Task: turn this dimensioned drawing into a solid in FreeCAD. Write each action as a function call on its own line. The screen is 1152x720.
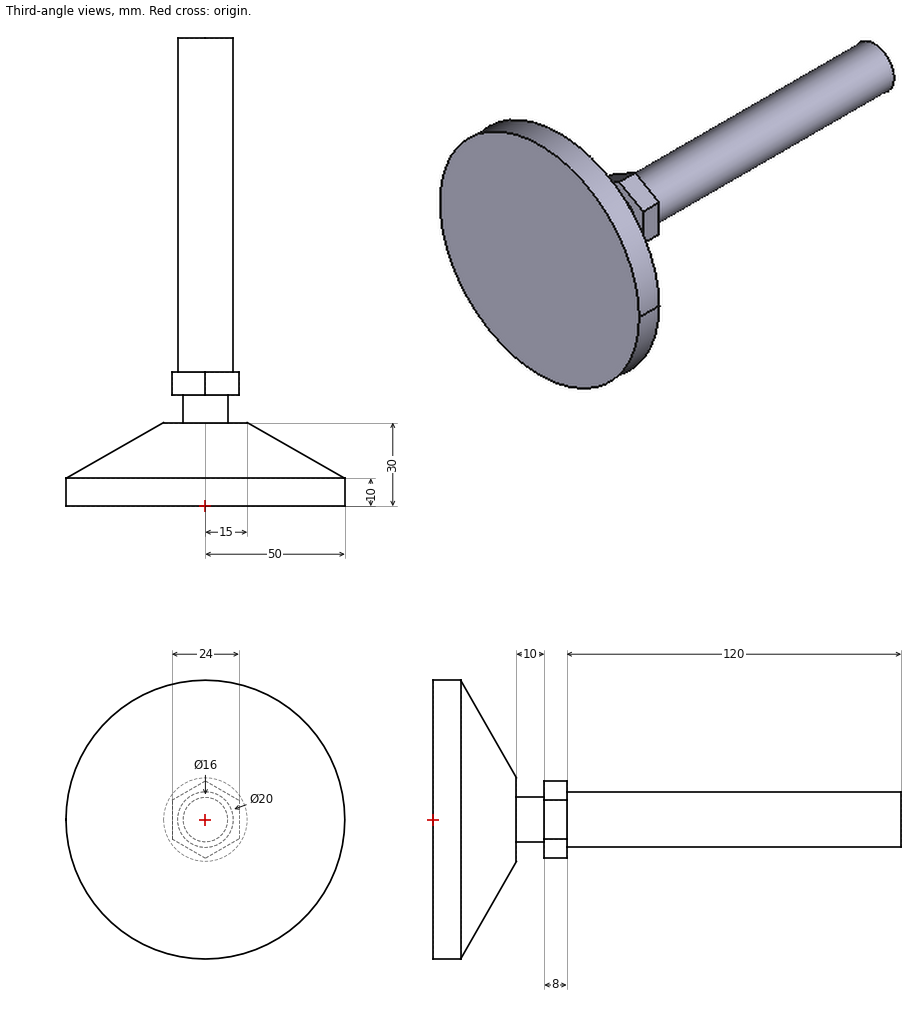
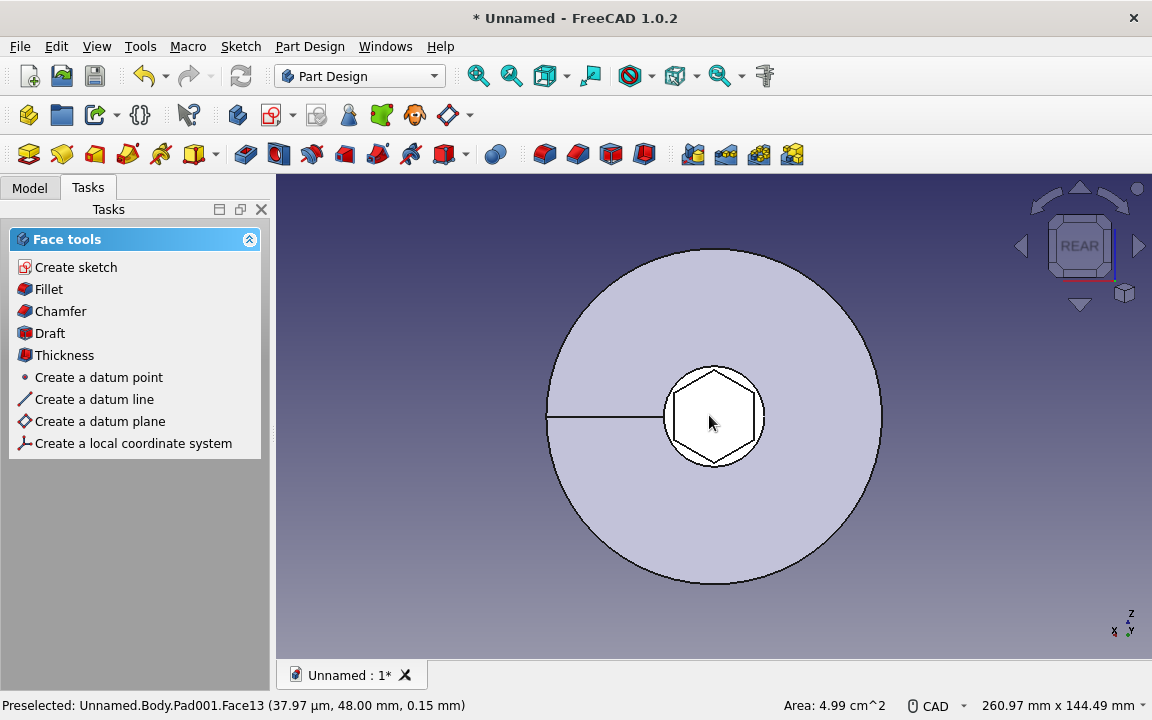
click(270, 116)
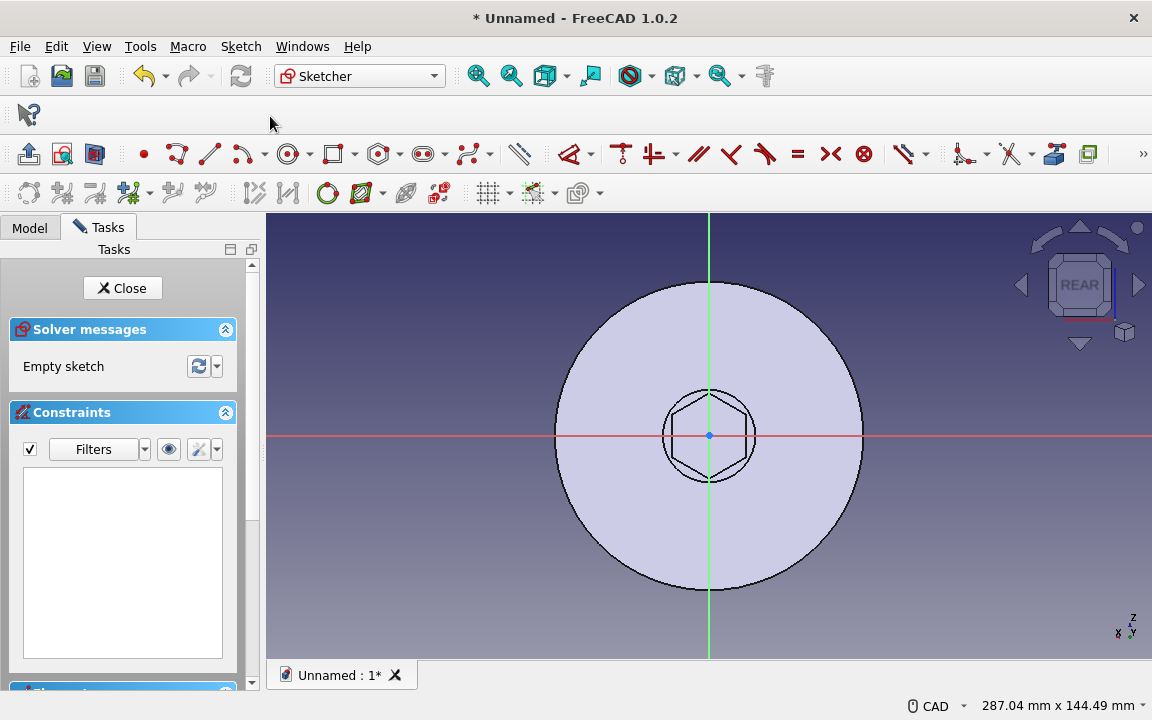
scroll(732, 436, up, 7)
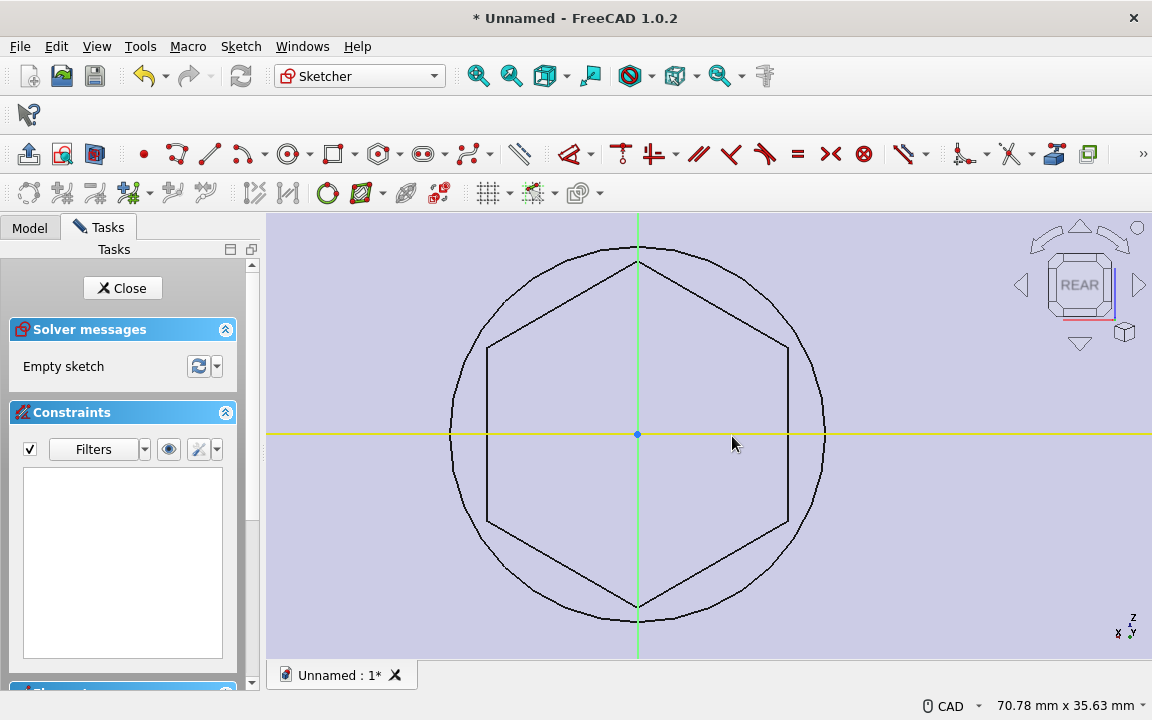
click(288, 154)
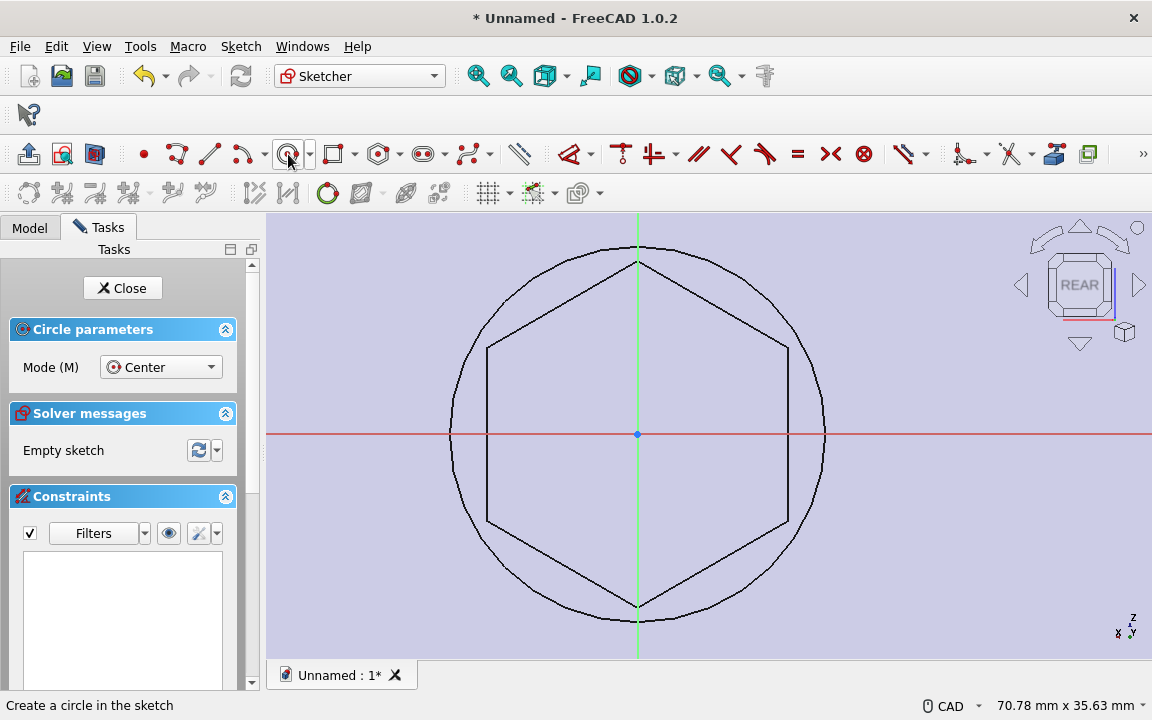
click(638, 434)
move(726, 346)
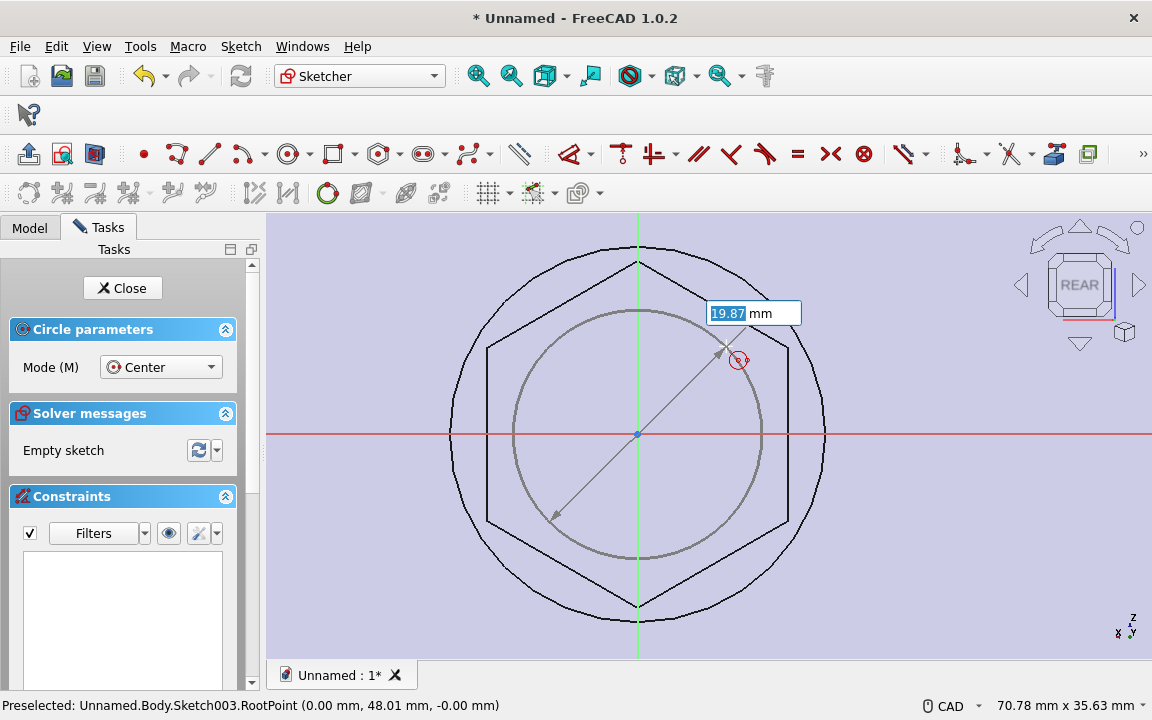
text(20)
key(Return)
key(Escape)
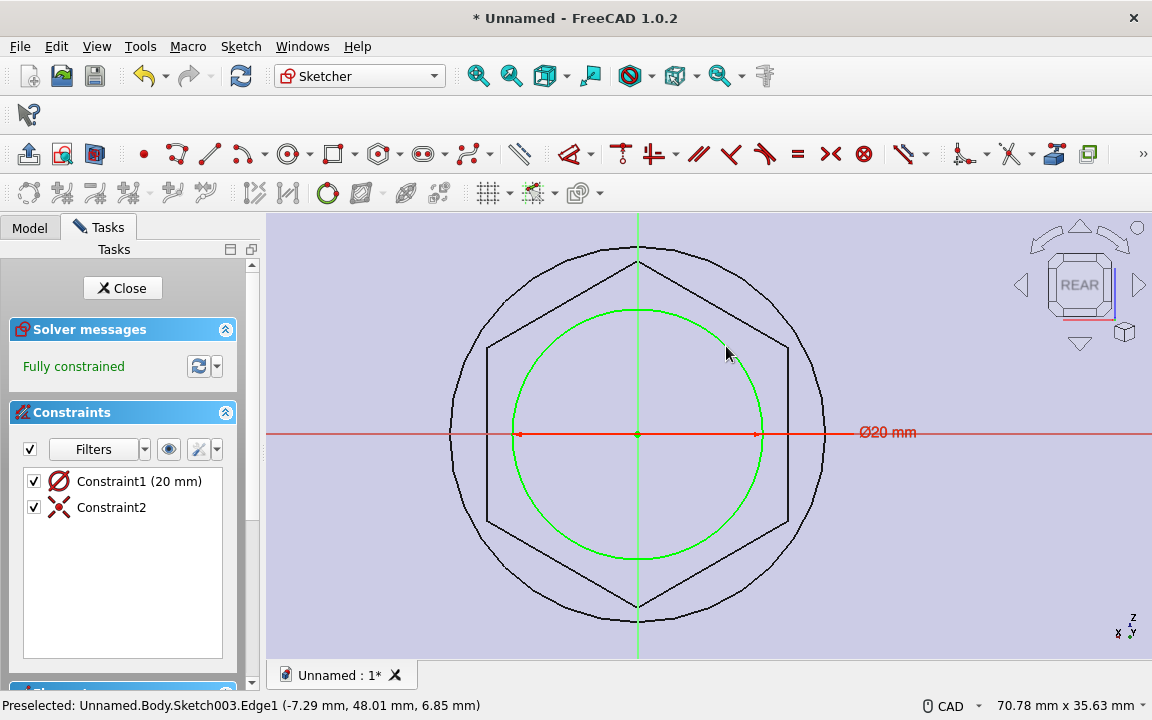
click(123, 288)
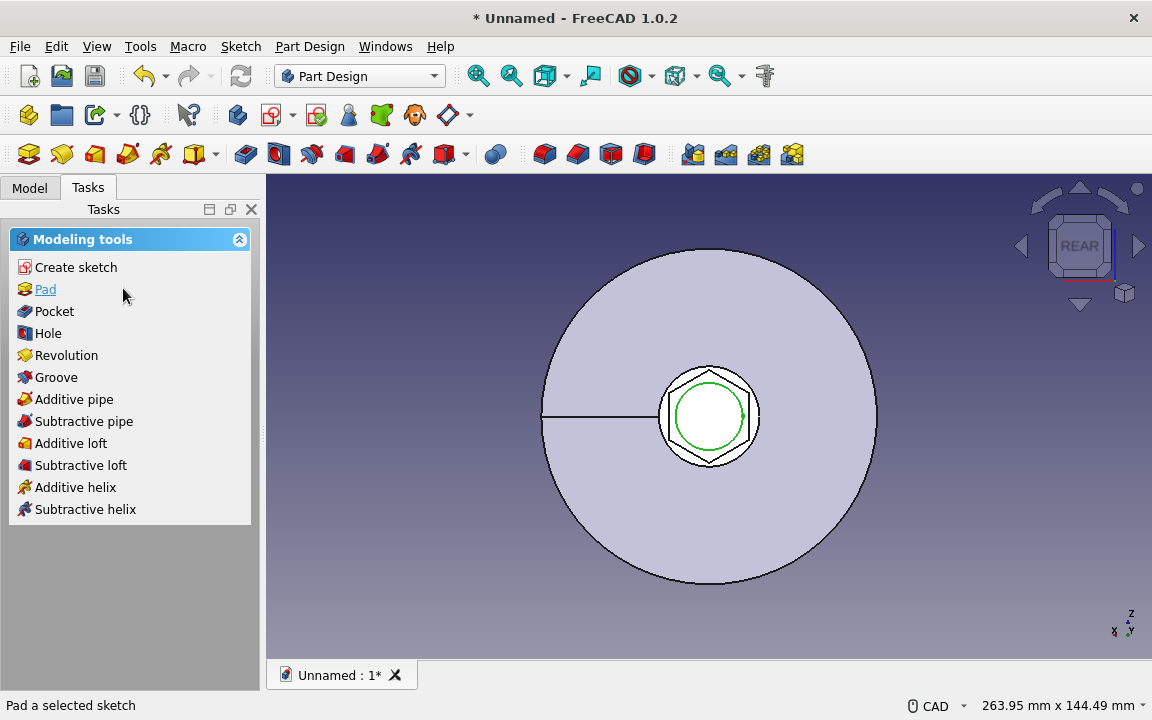
click(29, 154)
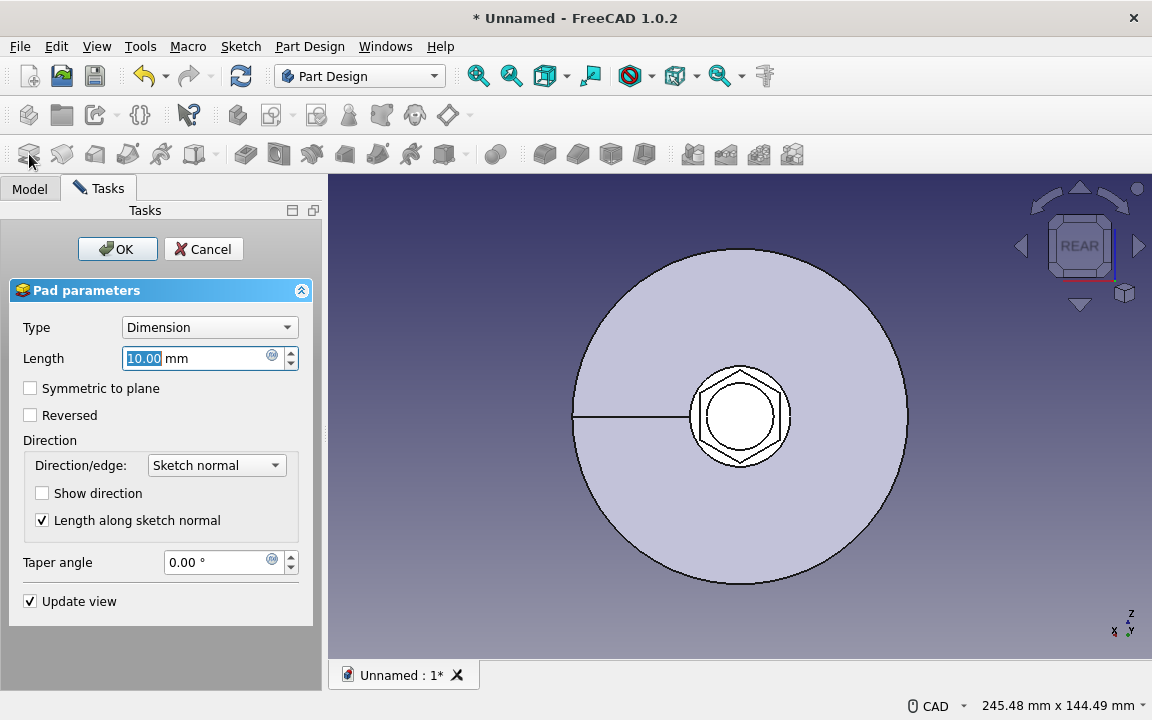
text(120)
key(Tab)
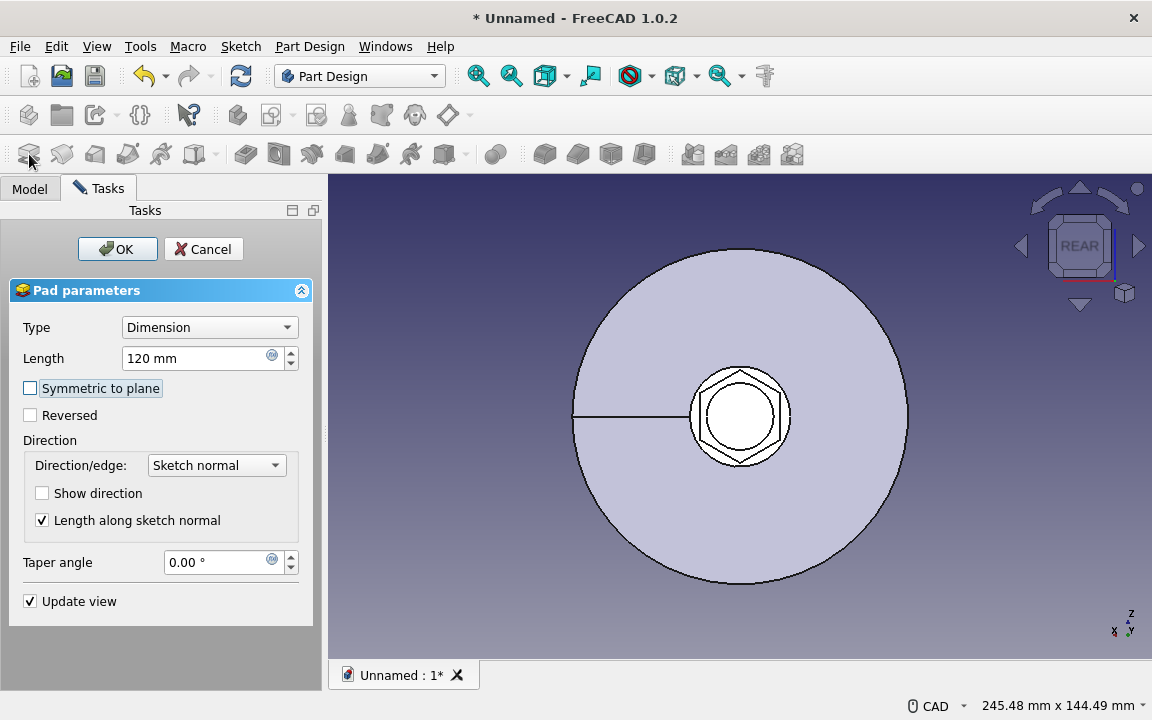
click(118, 249)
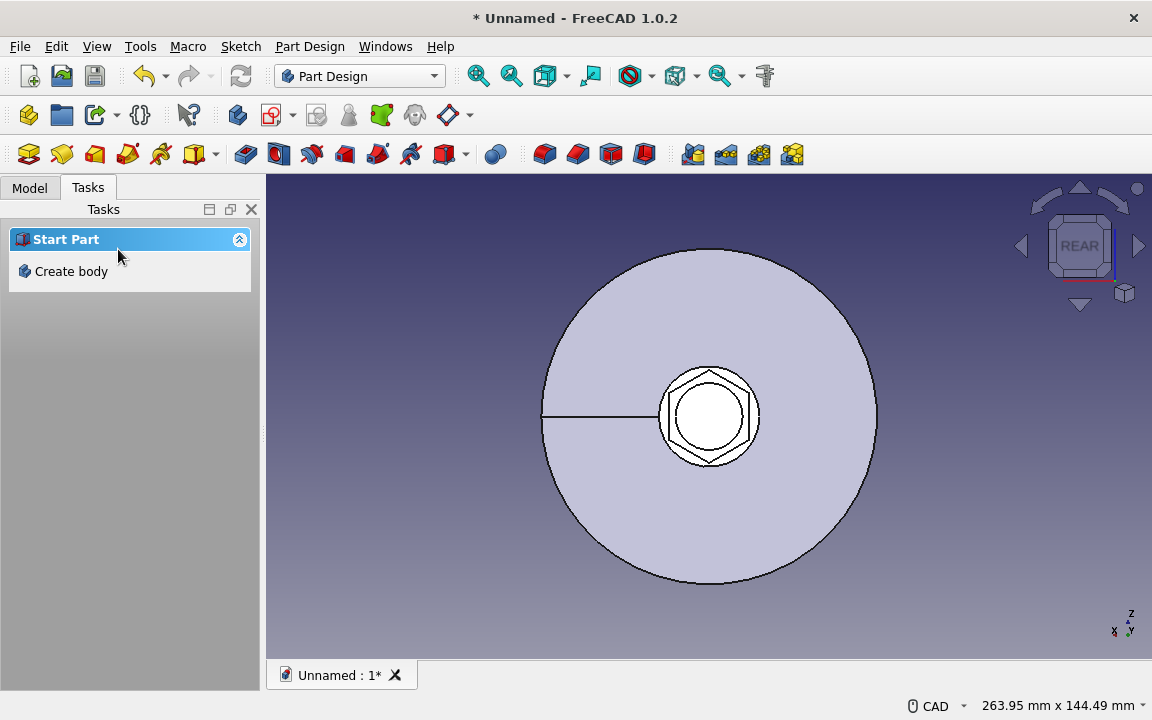
key(0)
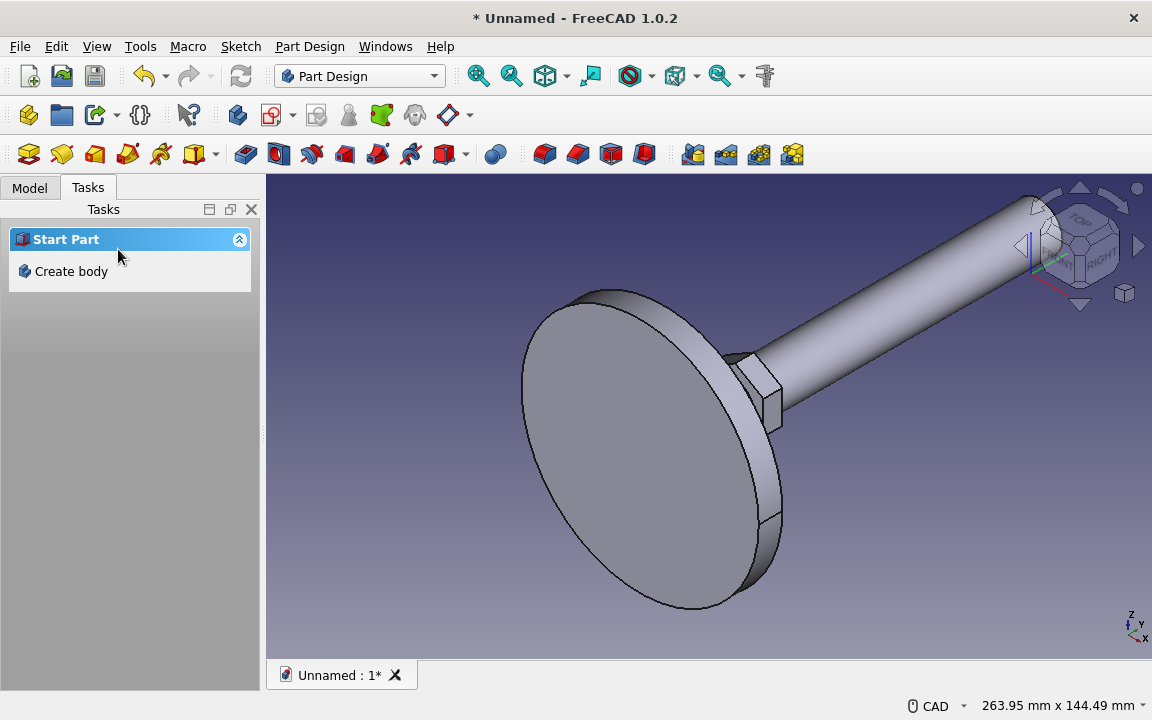
key(v)
key(f)